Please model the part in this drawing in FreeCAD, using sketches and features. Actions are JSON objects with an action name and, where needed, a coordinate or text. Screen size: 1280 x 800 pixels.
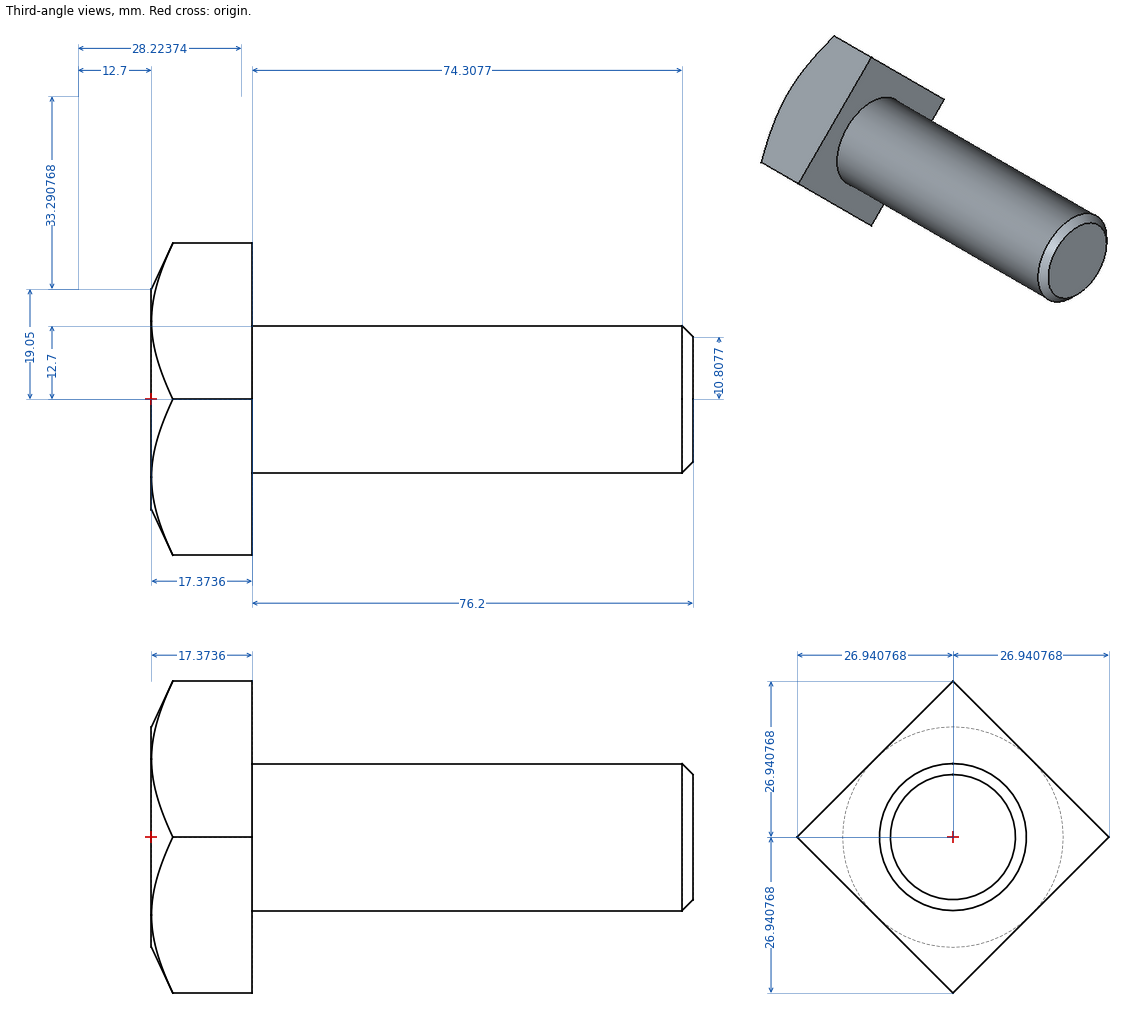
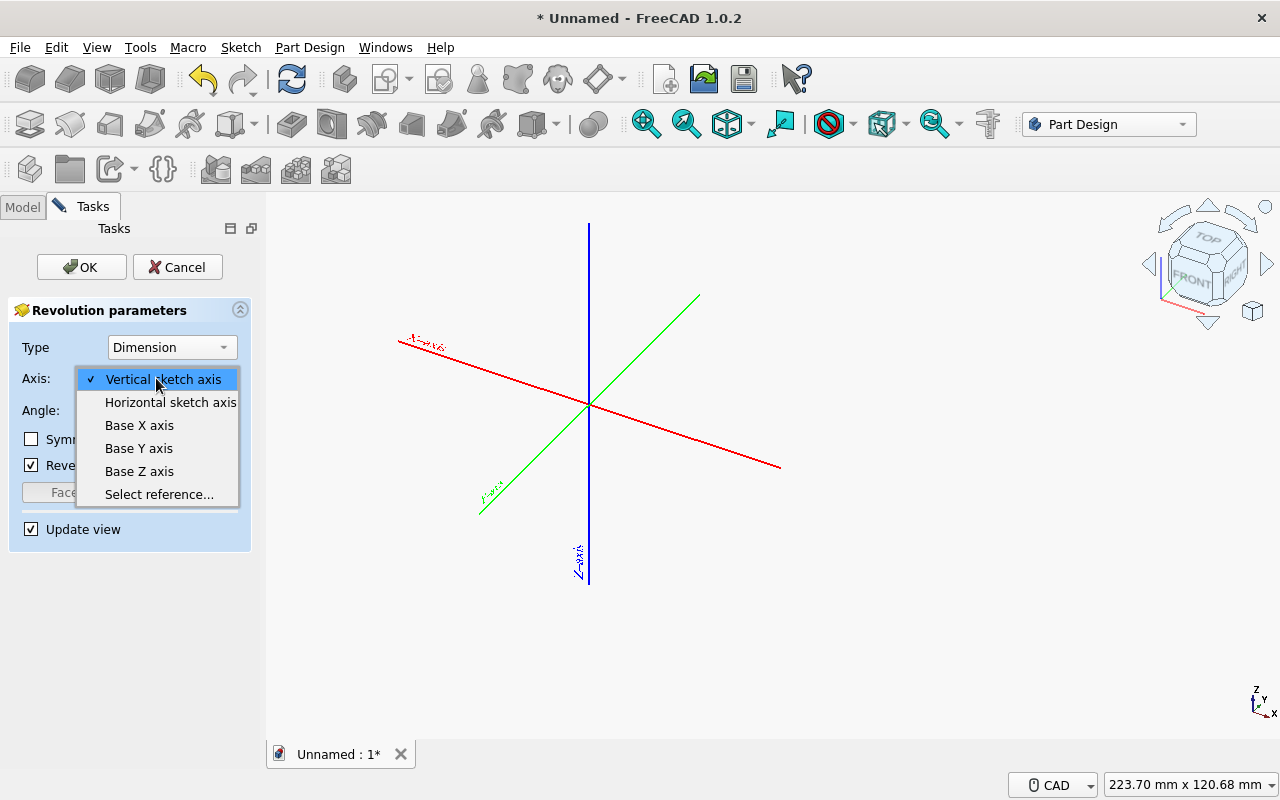
{"action": "left_click", "coordinate": [156, 402]}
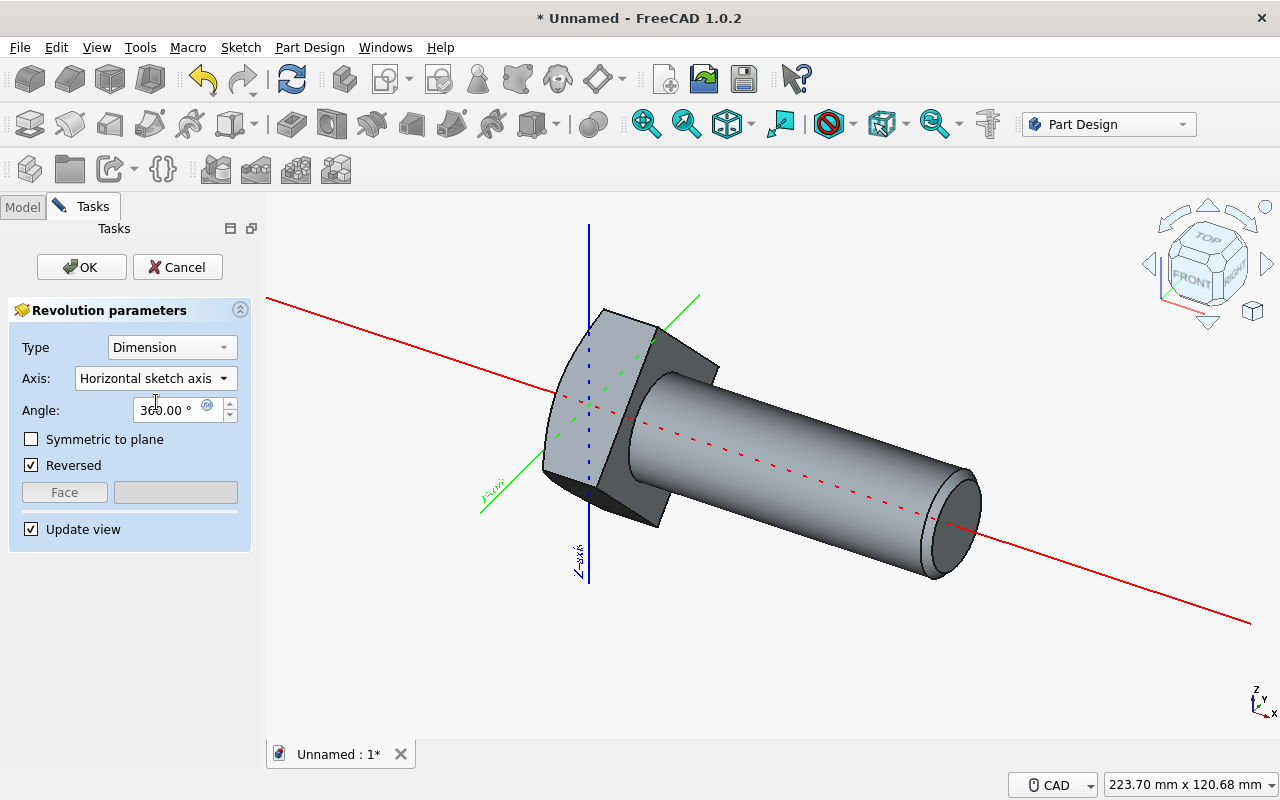
{"action": "left_click", "coordinate": [82, 267]}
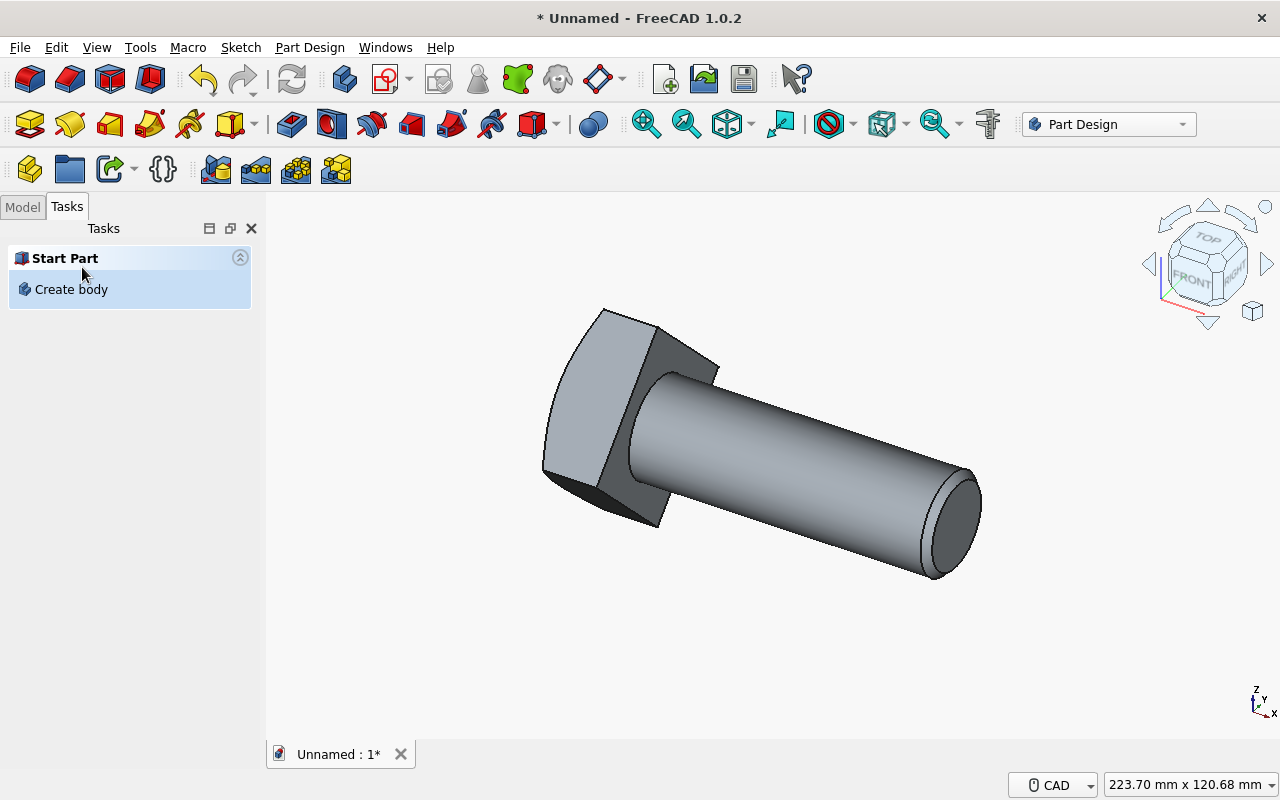
{"action": "key", "text": "0"}